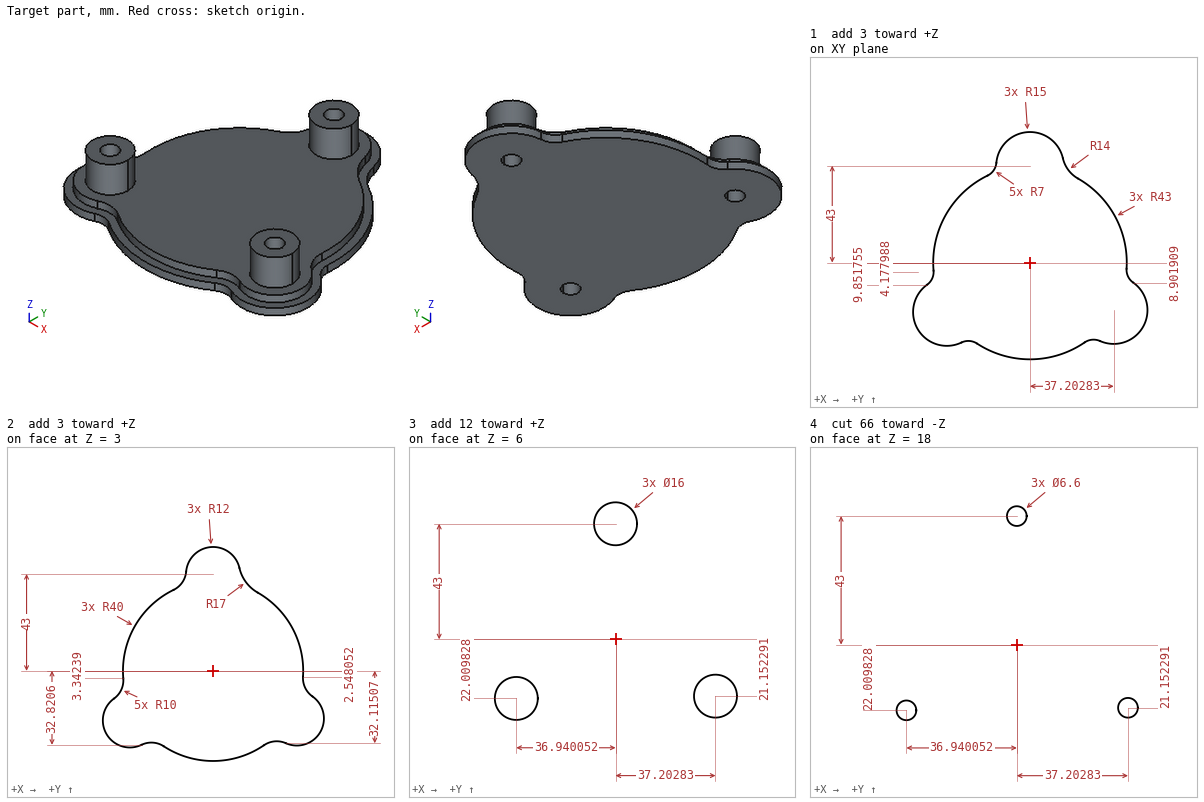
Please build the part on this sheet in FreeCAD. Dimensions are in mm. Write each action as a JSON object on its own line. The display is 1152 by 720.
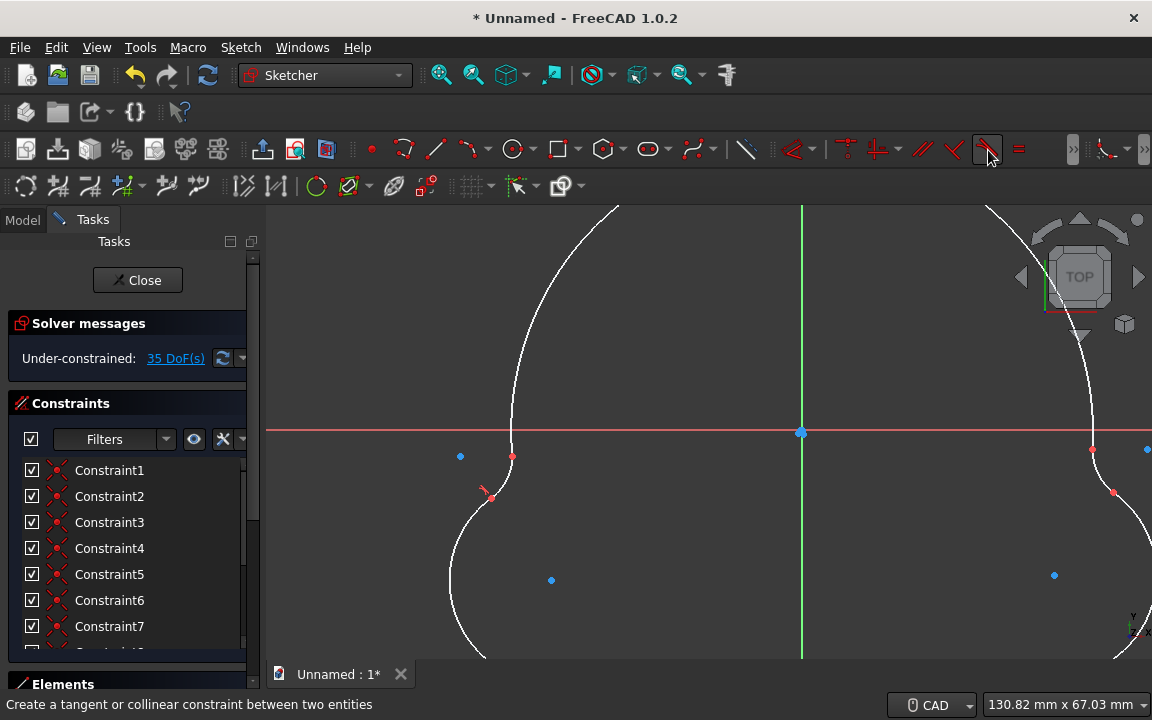
{"action": "left_click", "coordinate": [502, 488]}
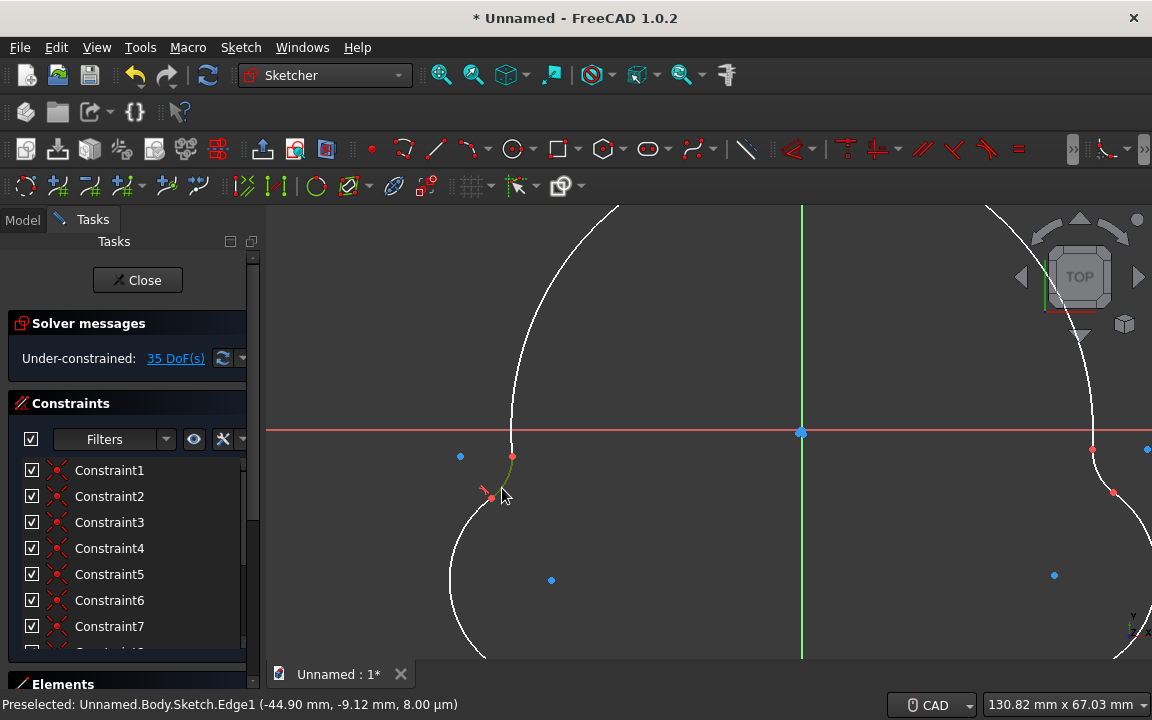
{"action": "left_click", "coordinate": [522, 352]}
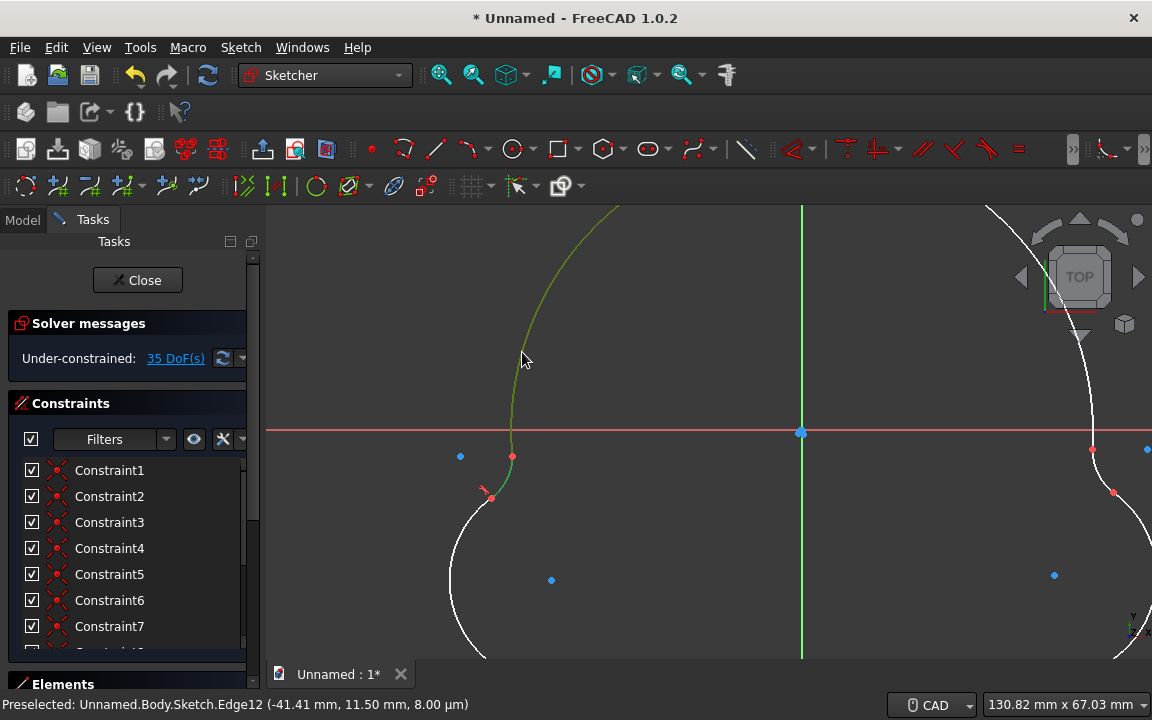
{"action": "left_click", "coordinate": [988, 150]}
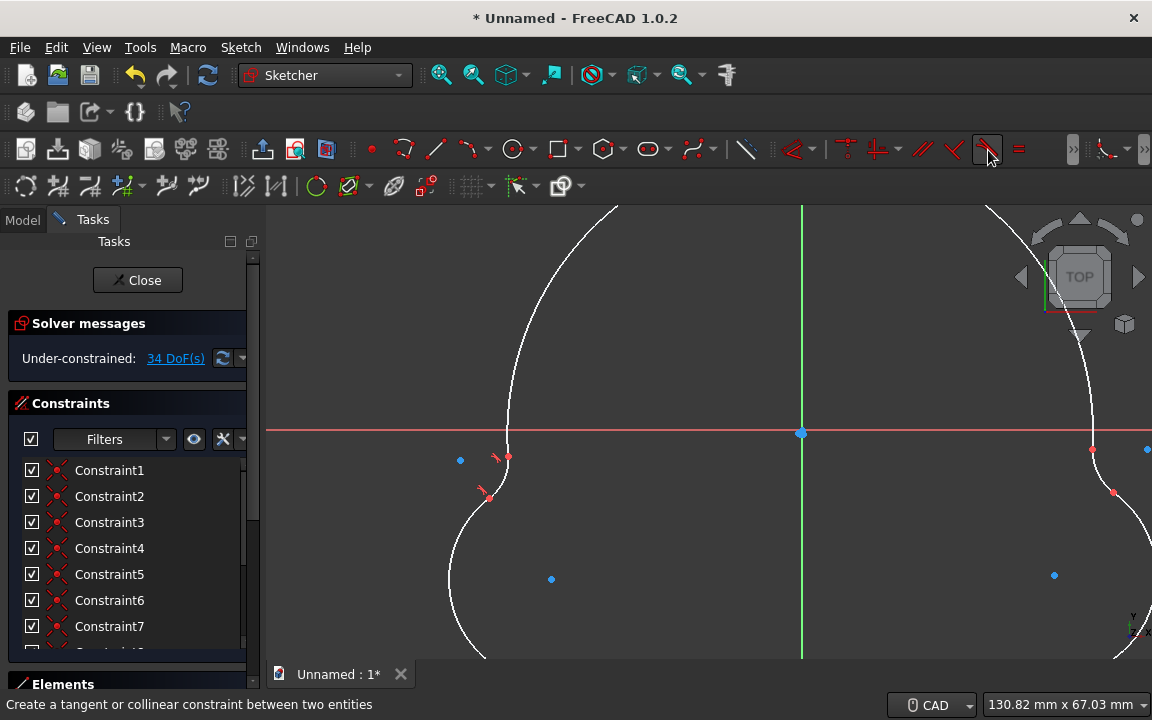
{"action": "left_click", "coordinate": [449, 576]}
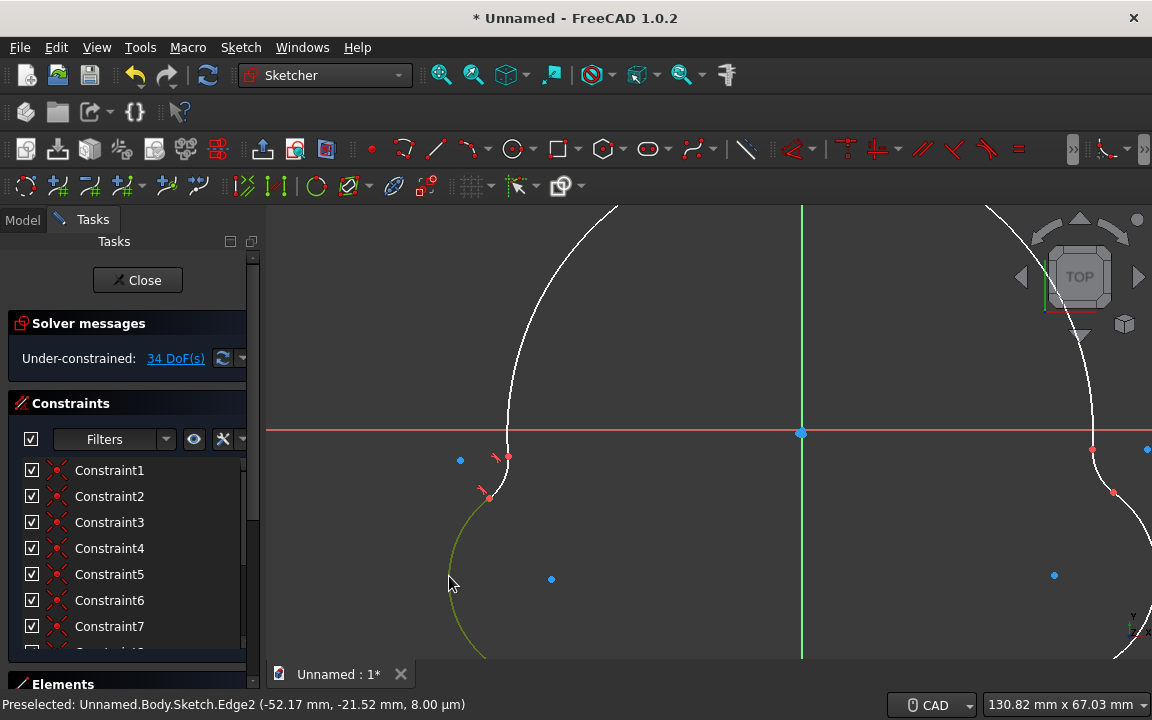
{"action": "scroll", "coordinate": [507, 475], "scroll_direction": "down", "scroll_amount": 4}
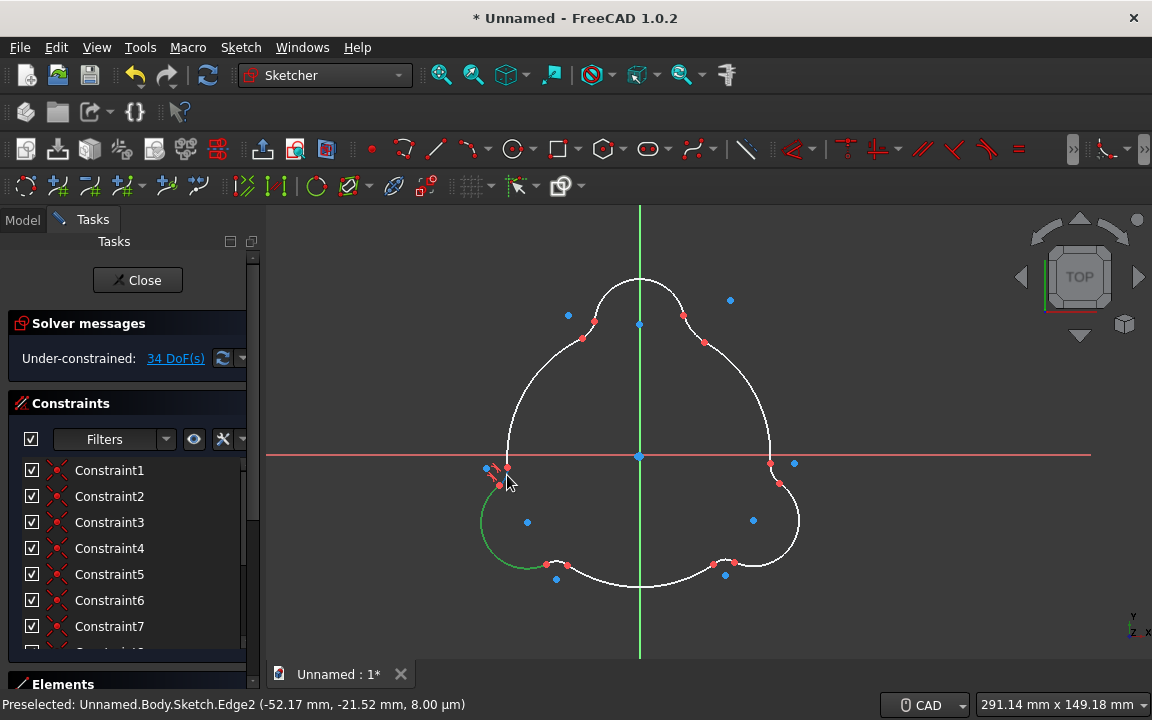
{"action": "scroll", "coordinate": [562, 562], "scroll_direction": "up", "scroll_amount": 4}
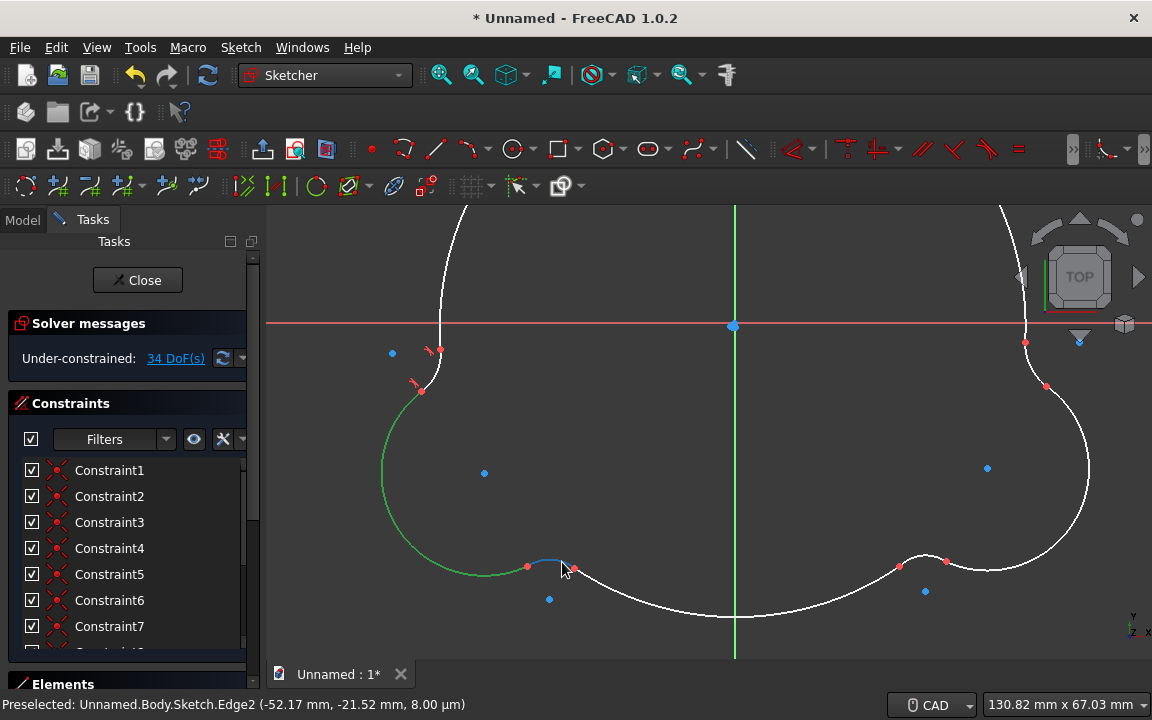
{"action": "left_click", "coordinate": [561, 561]}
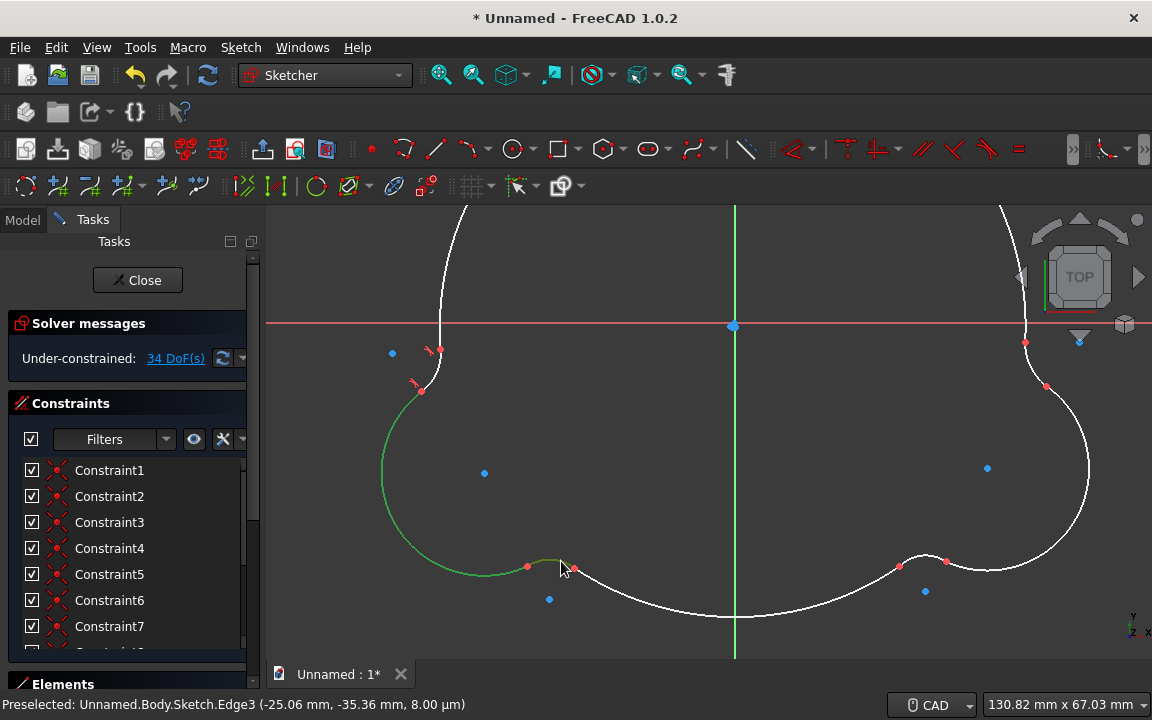
{"action": "left_click", "coordinate": [988, 150]}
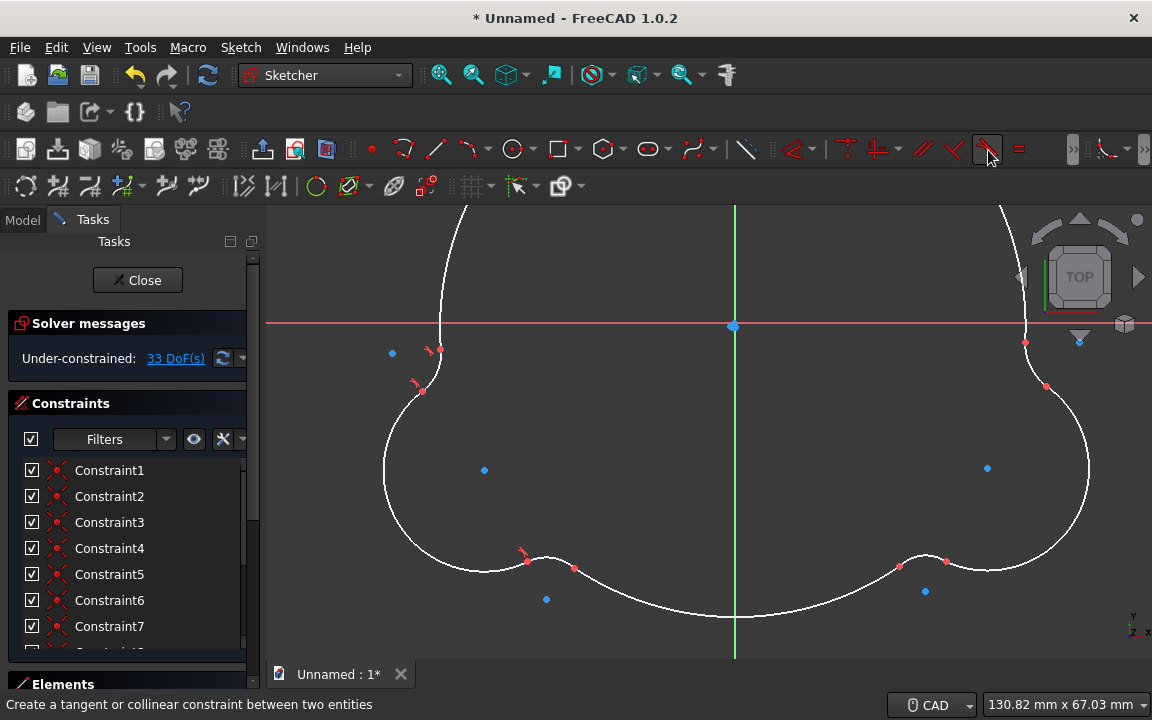
{"action": "left_click", "coordinate": [562, 560]}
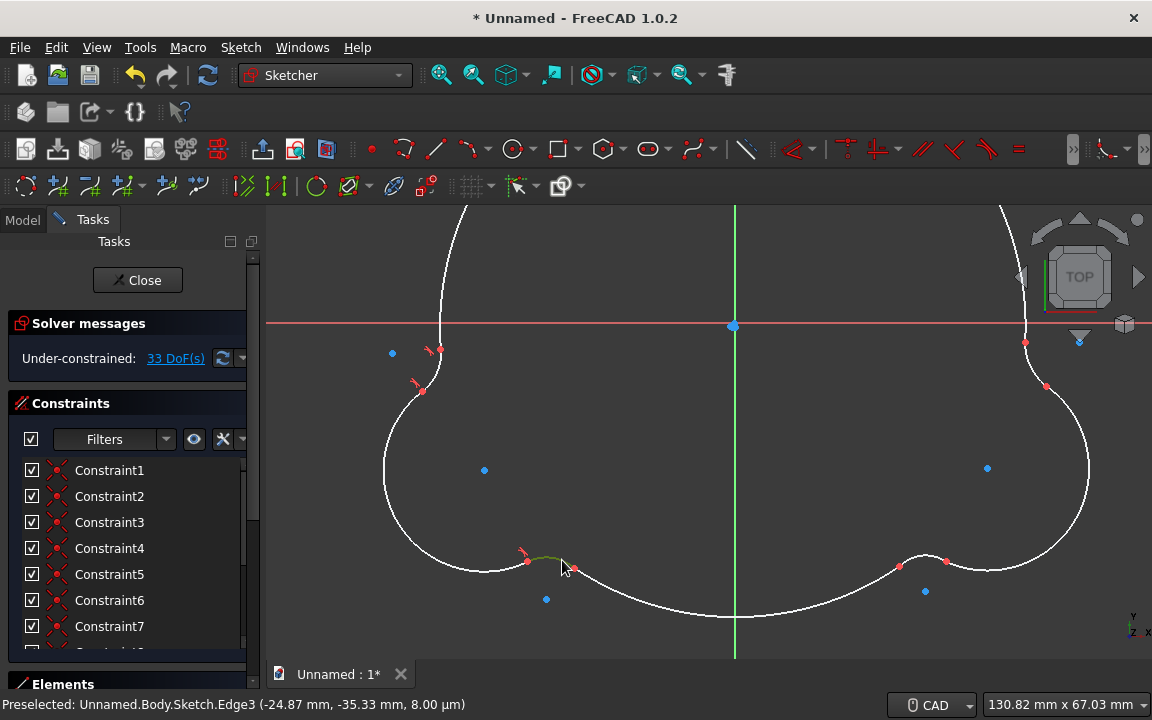
{"action": "left_click", "coordinate": [669, 609]}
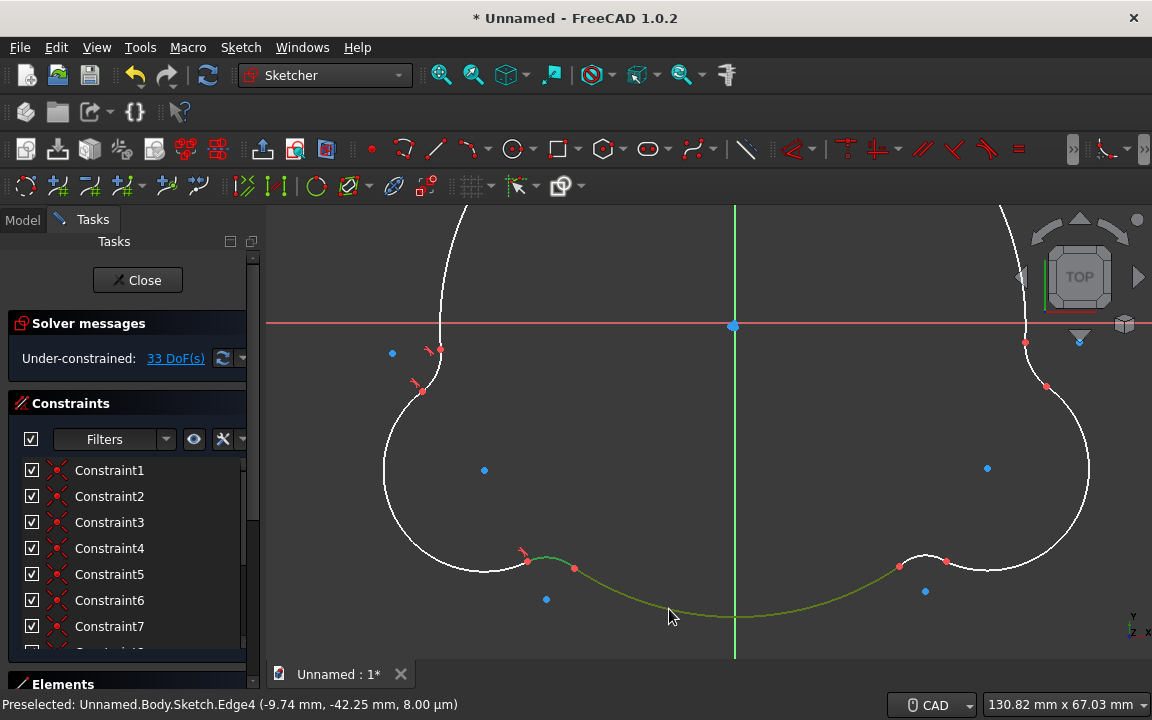
{"action": "left_click", "coordinate": [988, 150]}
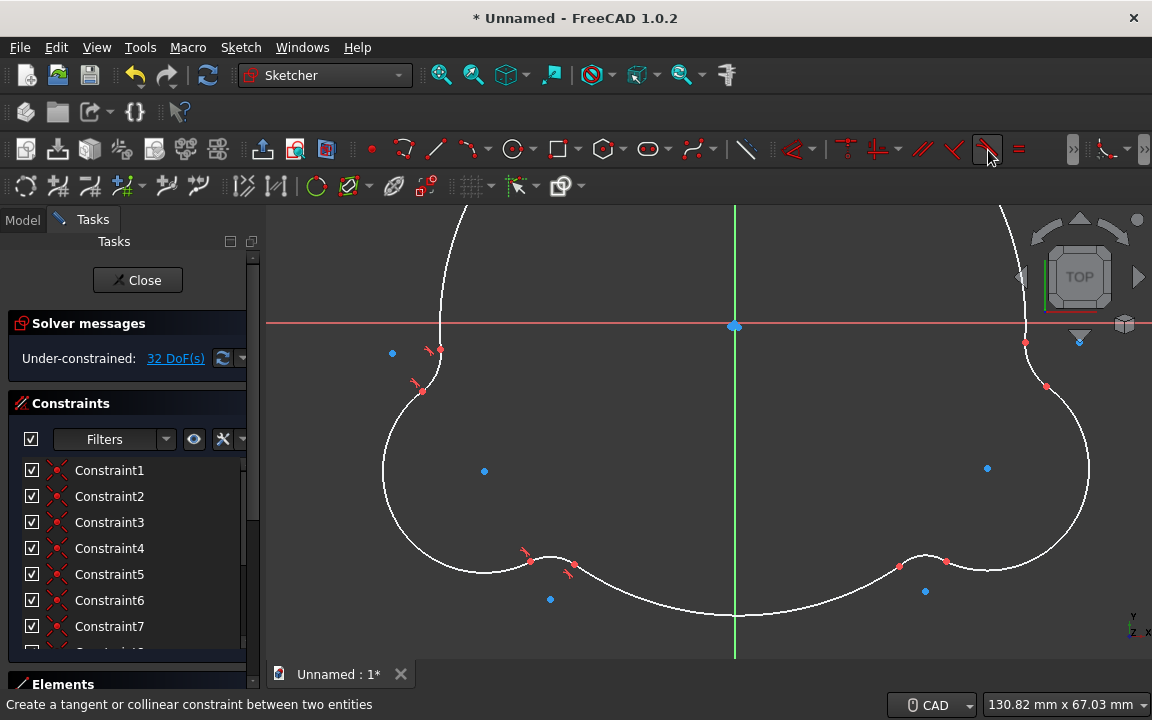
{"action": "left_click", "coordinate": [668, 607]}